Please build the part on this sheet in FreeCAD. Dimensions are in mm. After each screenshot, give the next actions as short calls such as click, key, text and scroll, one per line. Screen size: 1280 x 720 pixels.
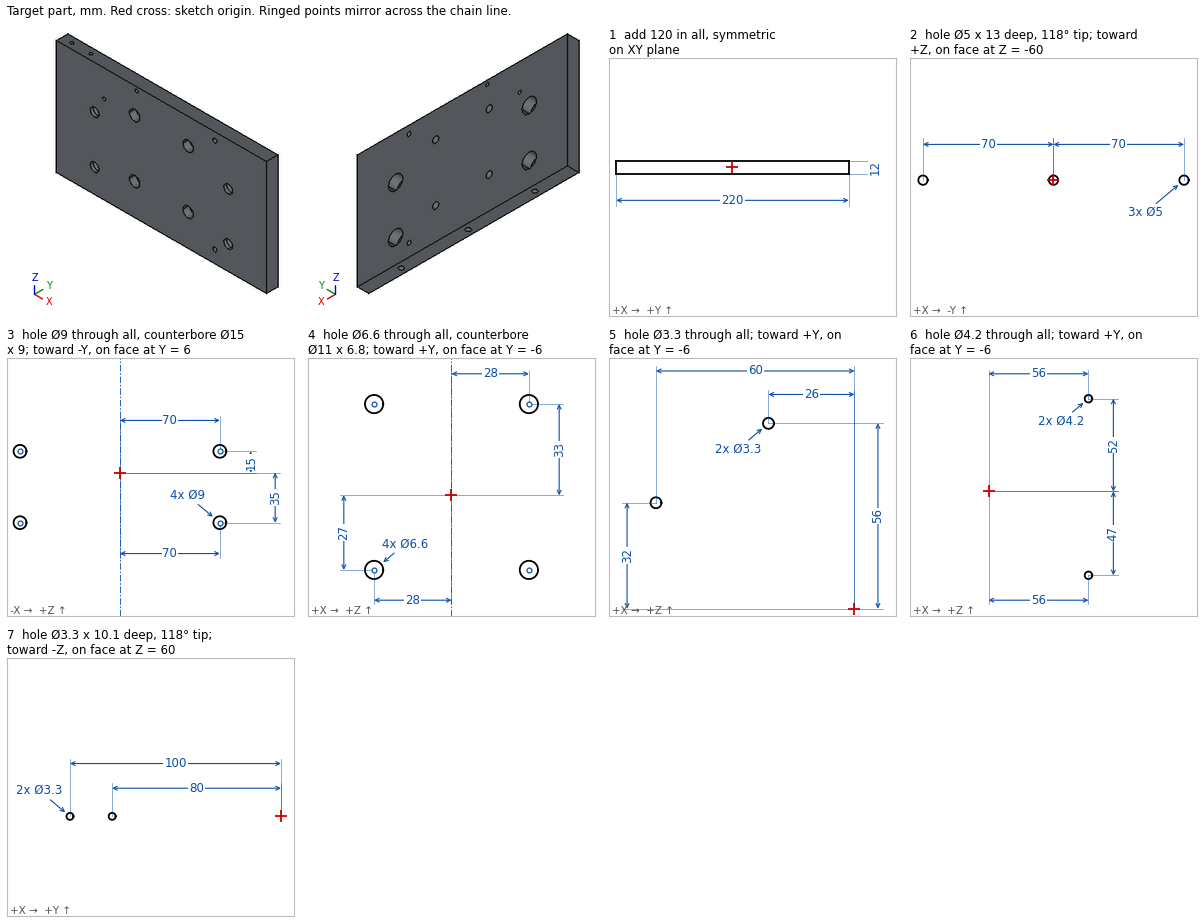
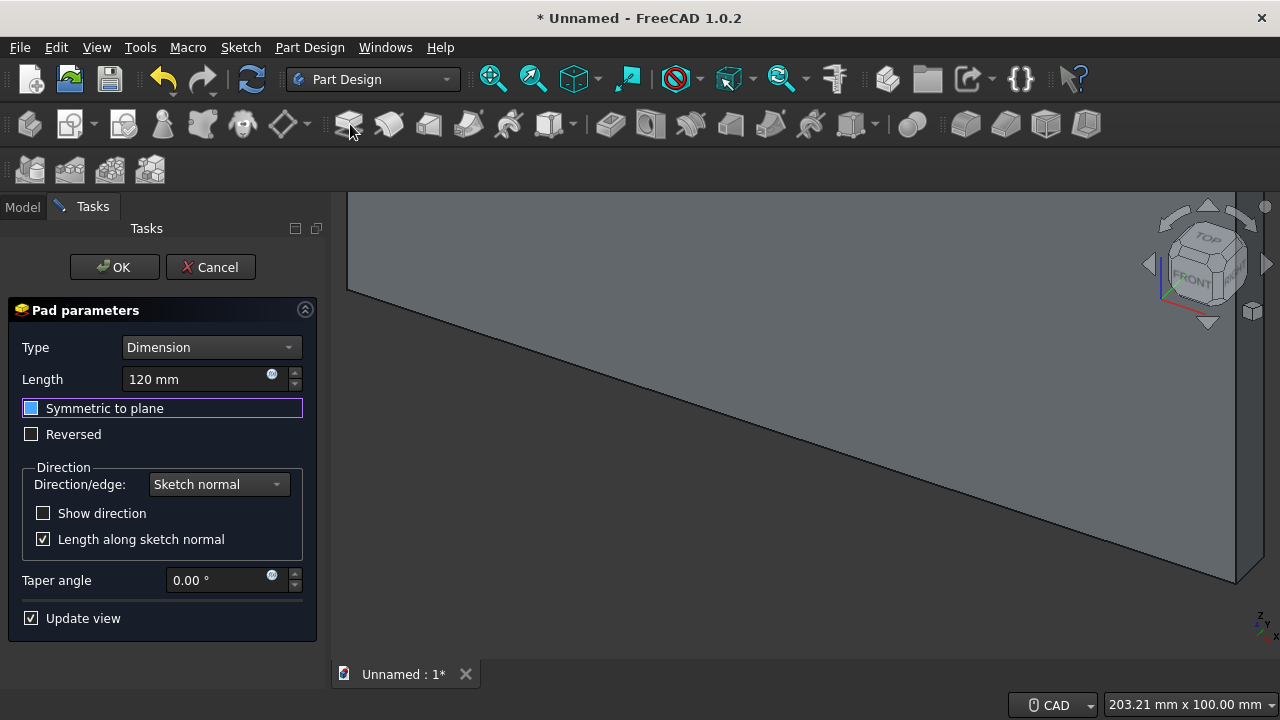
click(30, 408)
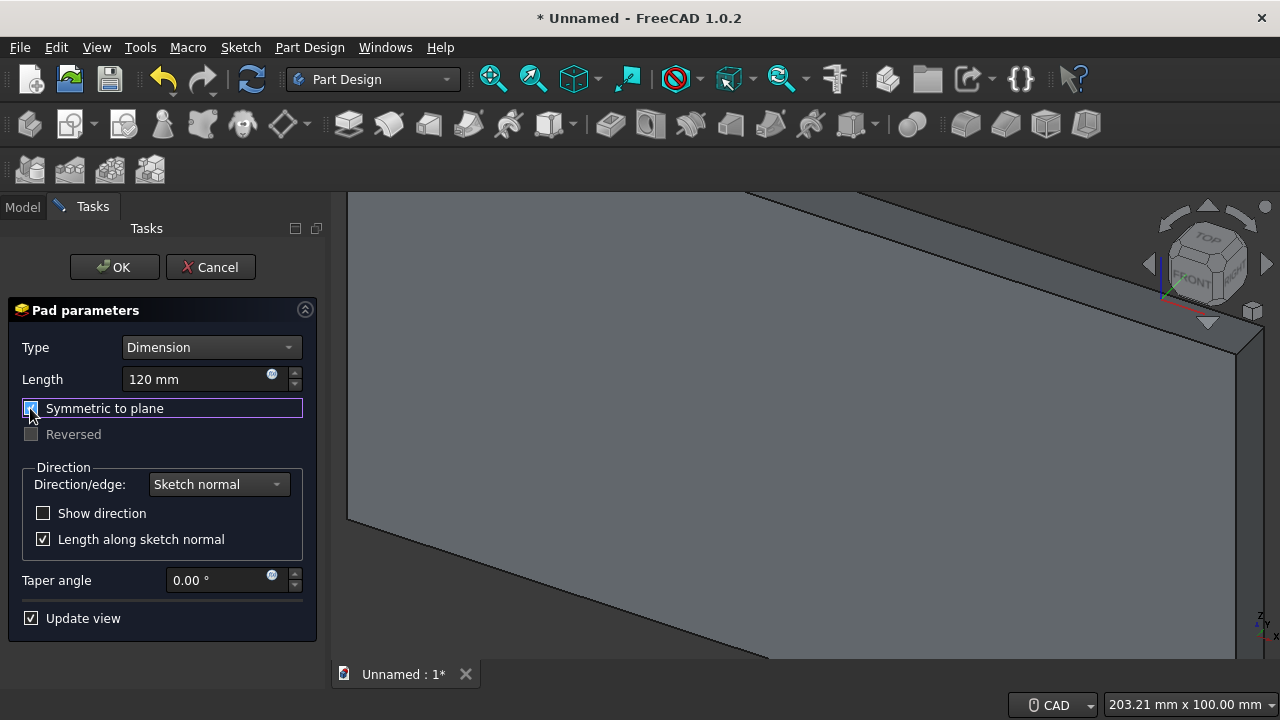
click(115, 267)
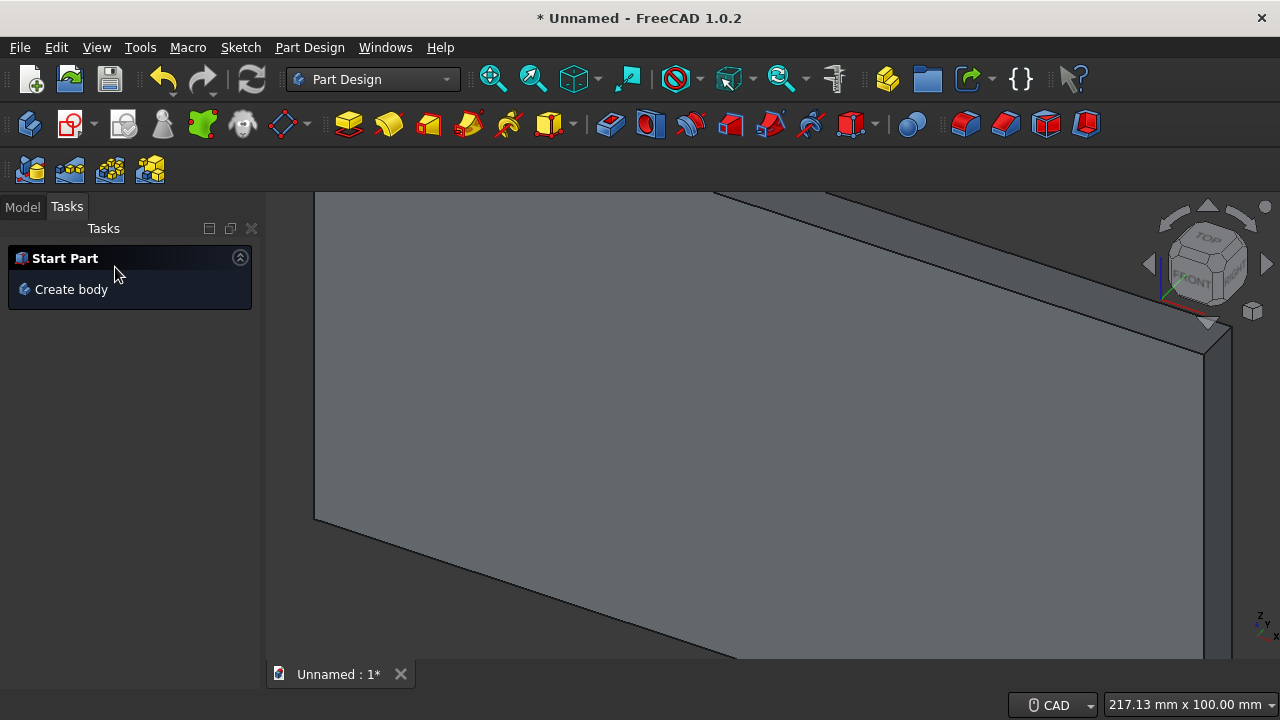
click(494, 80)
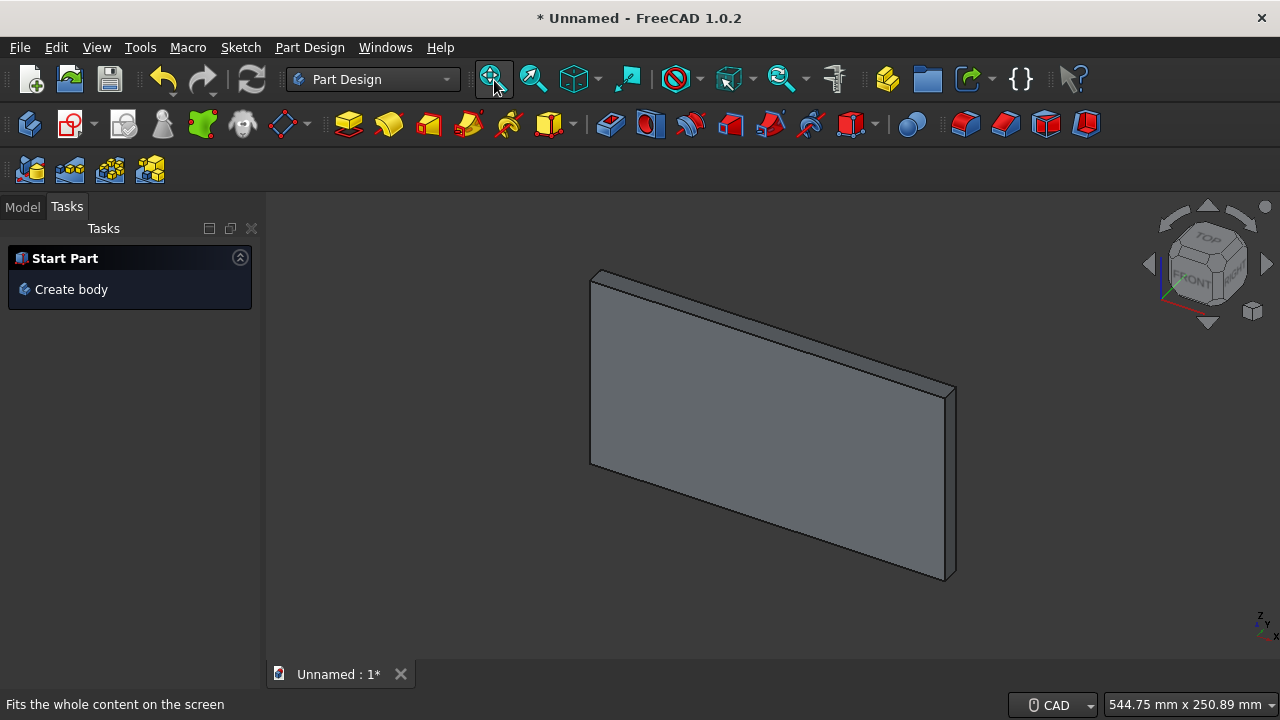
key(5)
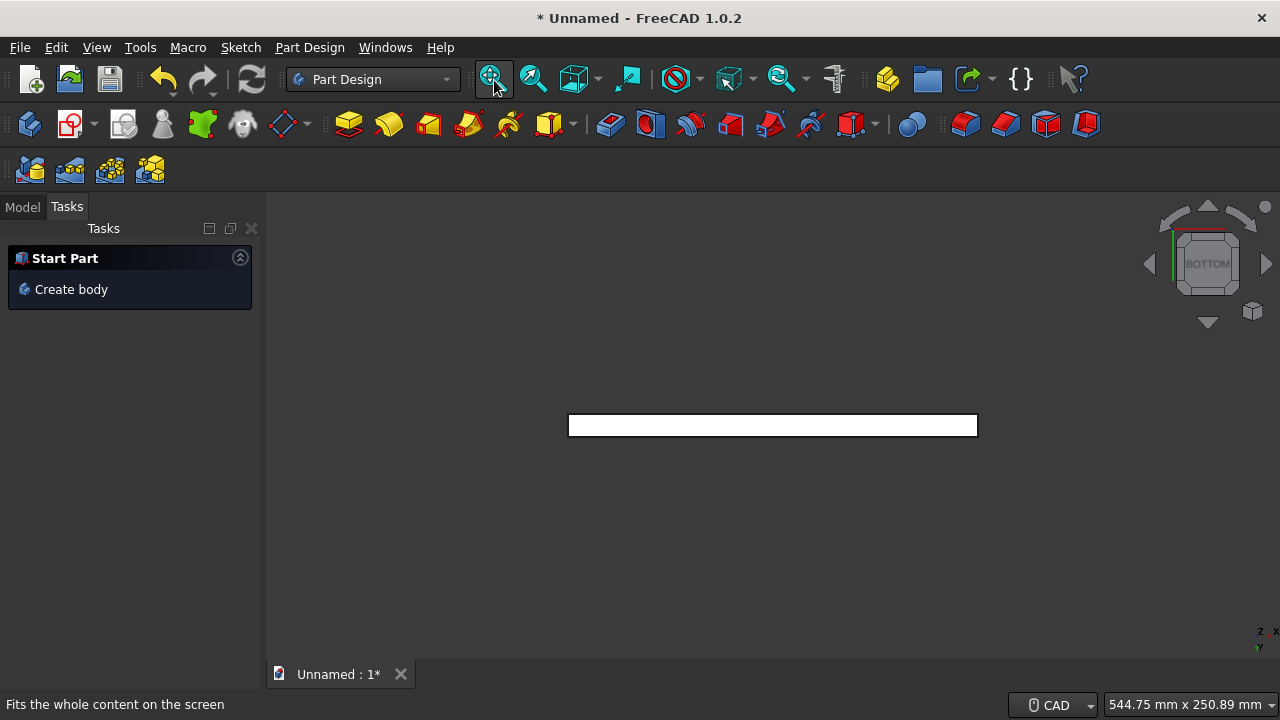
click(494, 80)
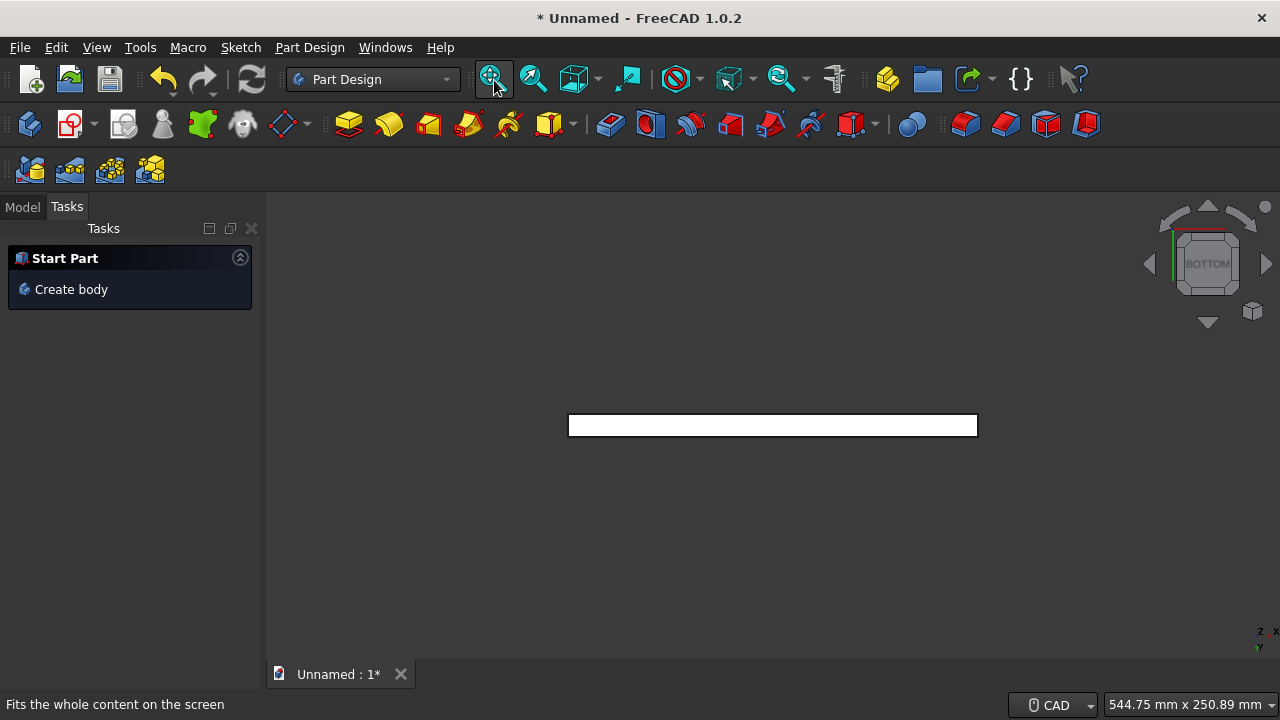
click(949, 424)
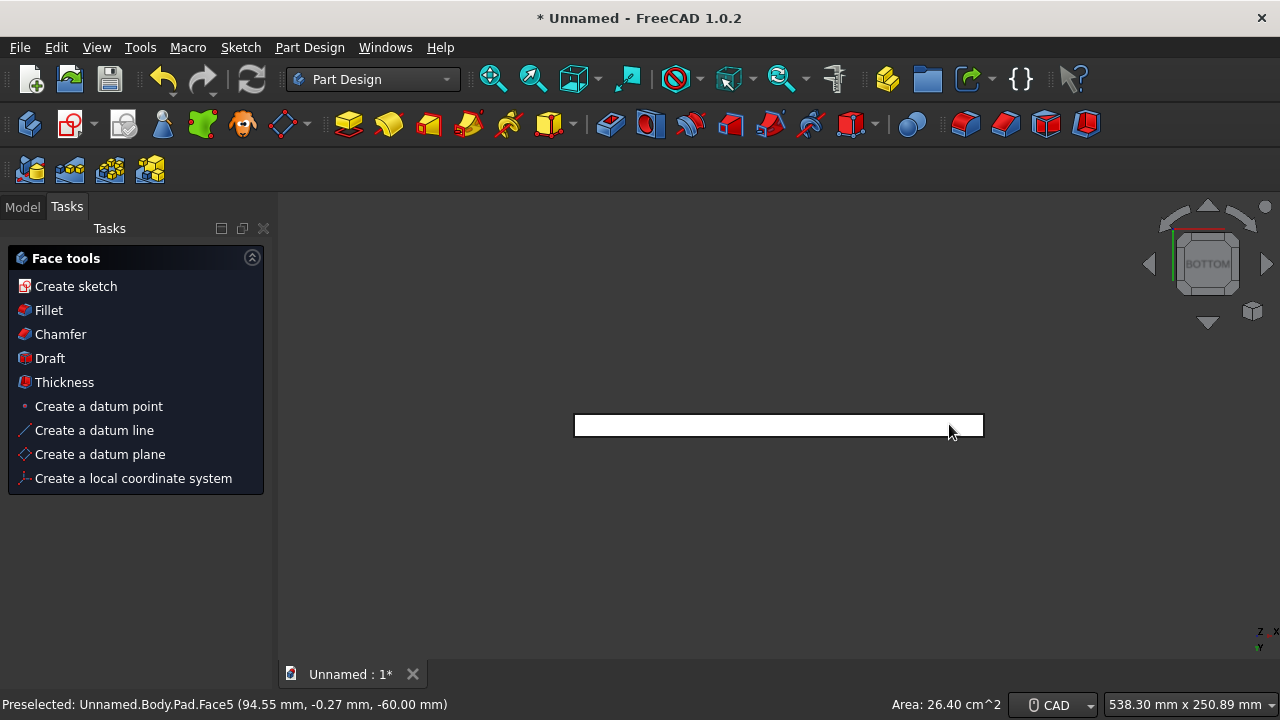
click(70, 124)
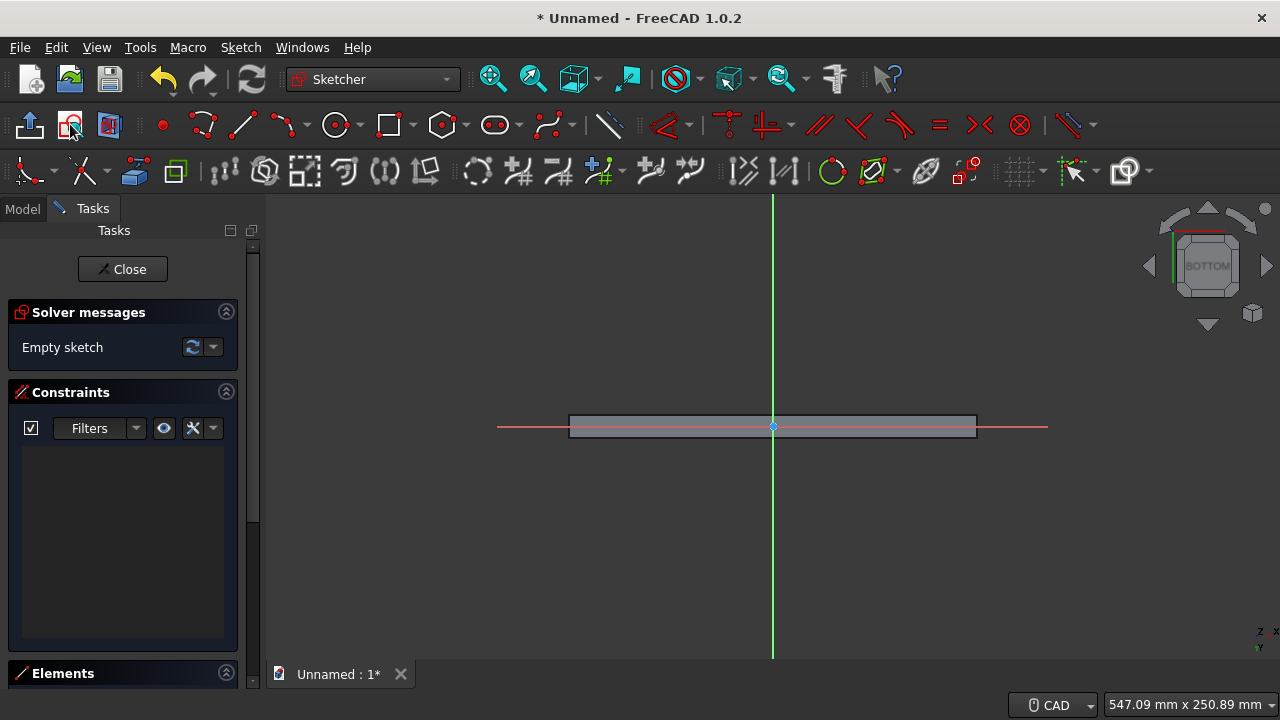
scroll(829, 426, up, 4)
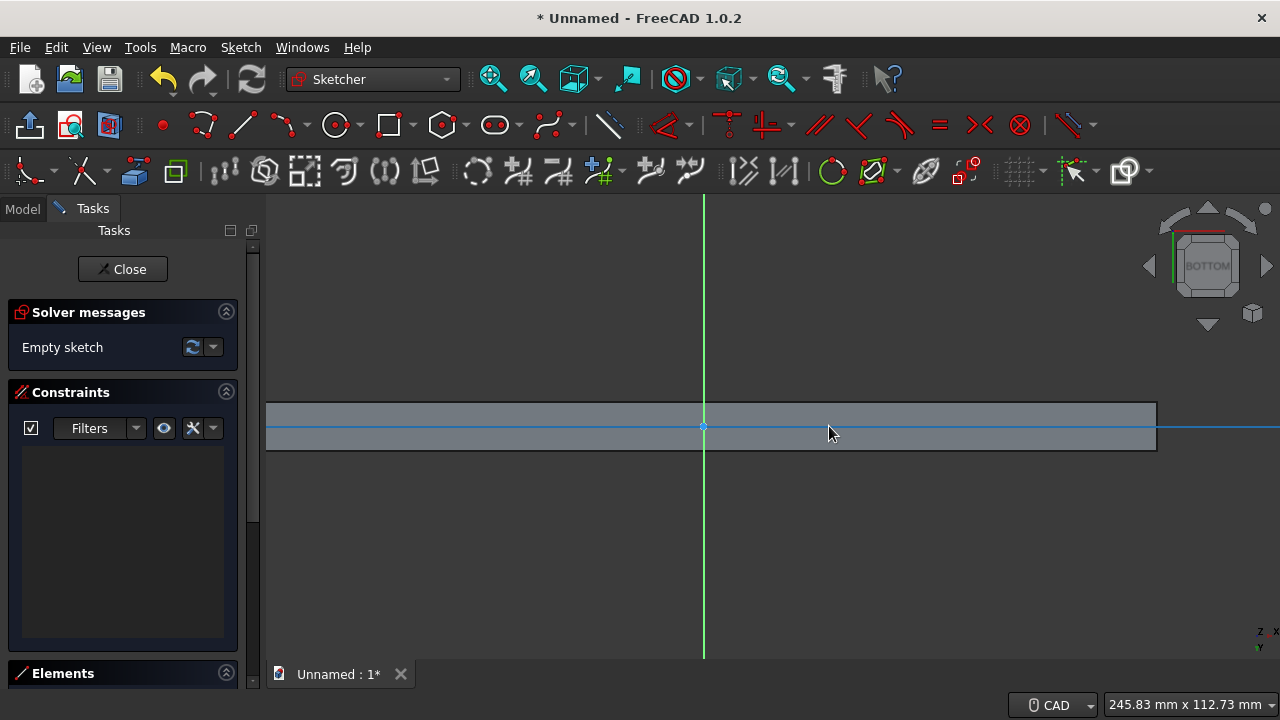
click(336, 126)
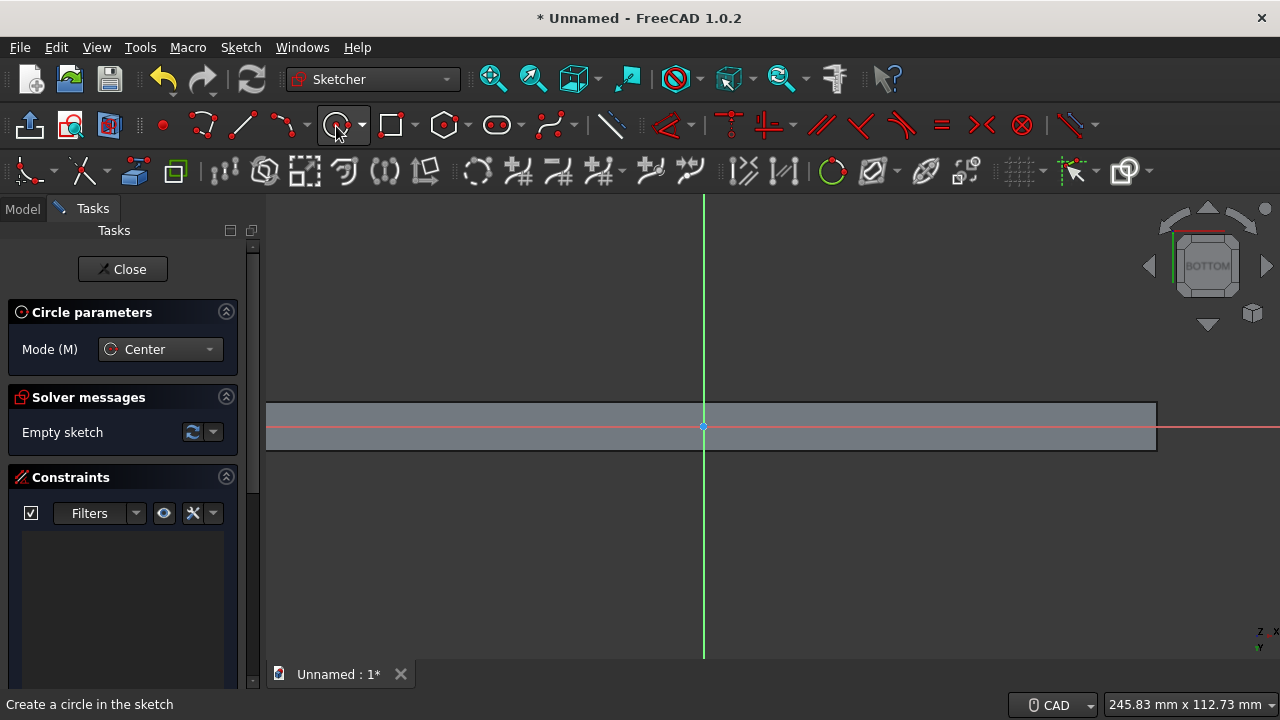
scroll(992, 426, up, 4)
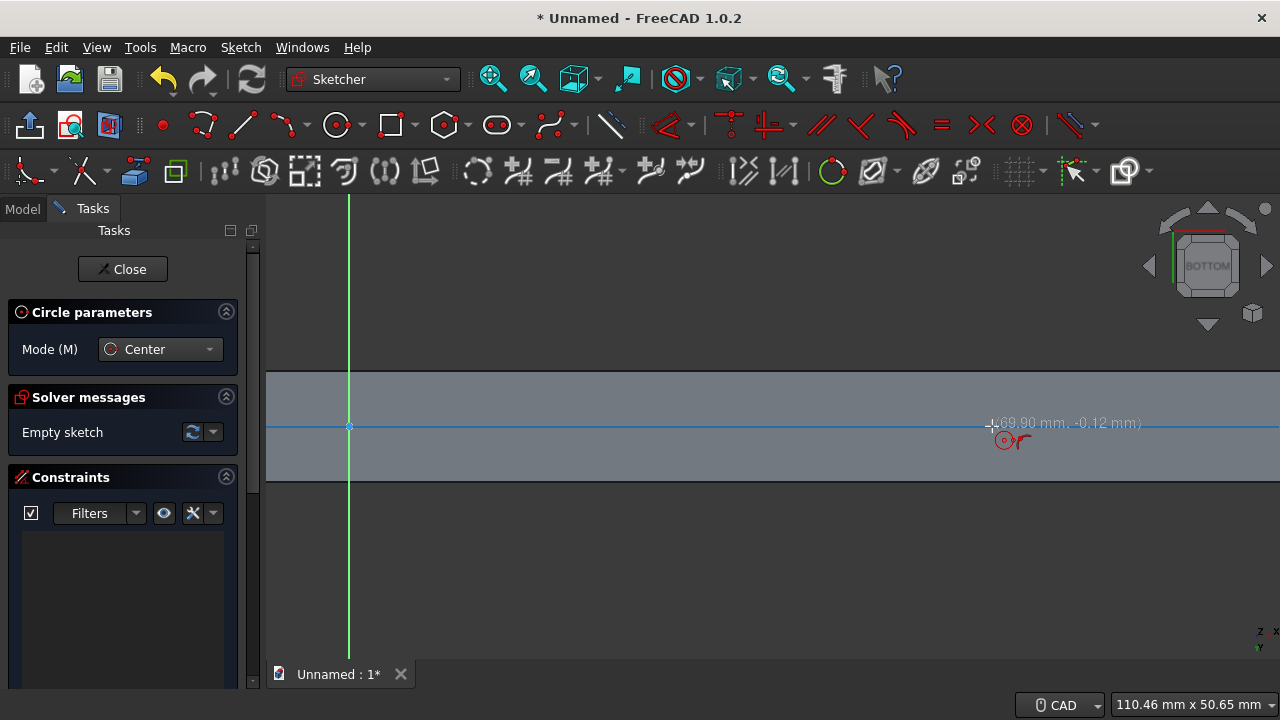
click(992, 426)
move(1008, 410)